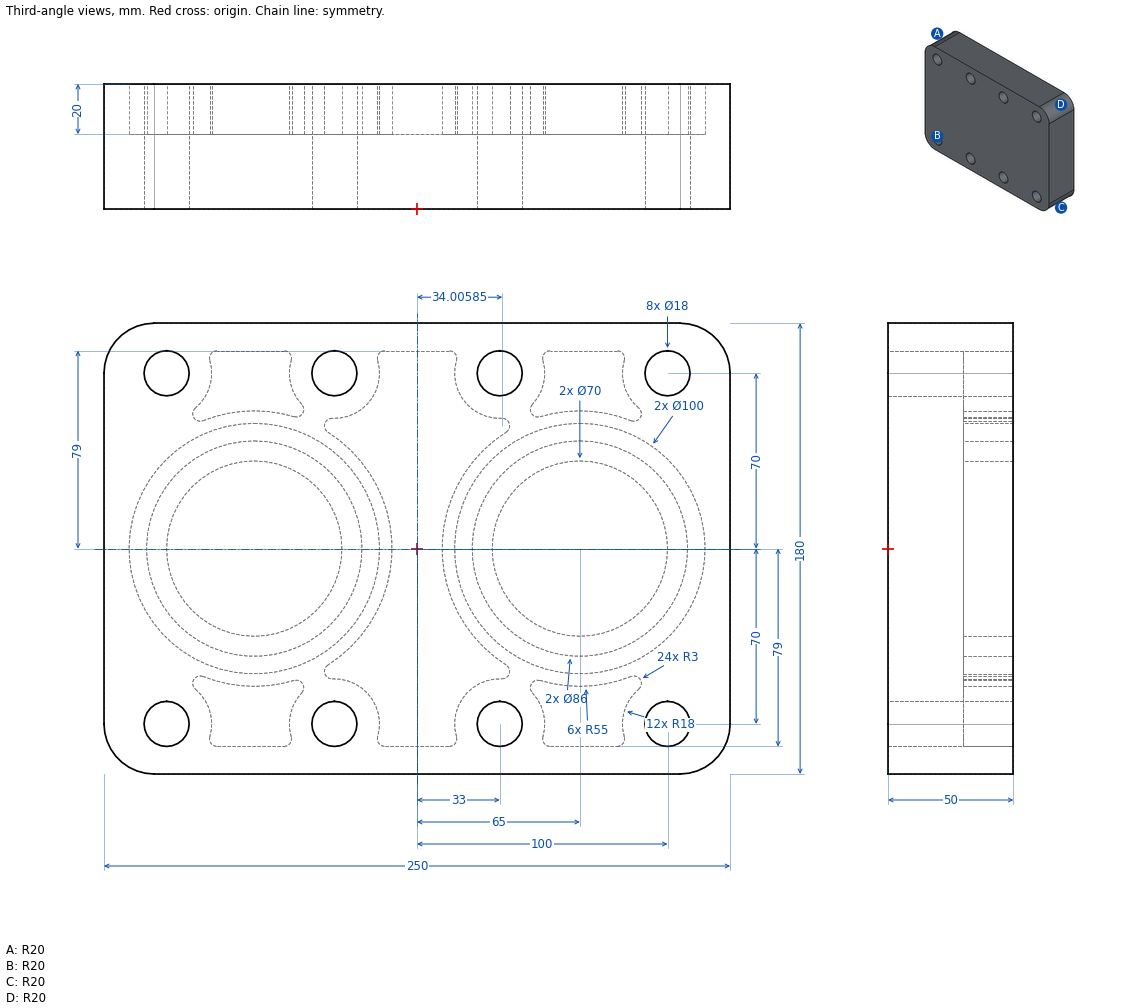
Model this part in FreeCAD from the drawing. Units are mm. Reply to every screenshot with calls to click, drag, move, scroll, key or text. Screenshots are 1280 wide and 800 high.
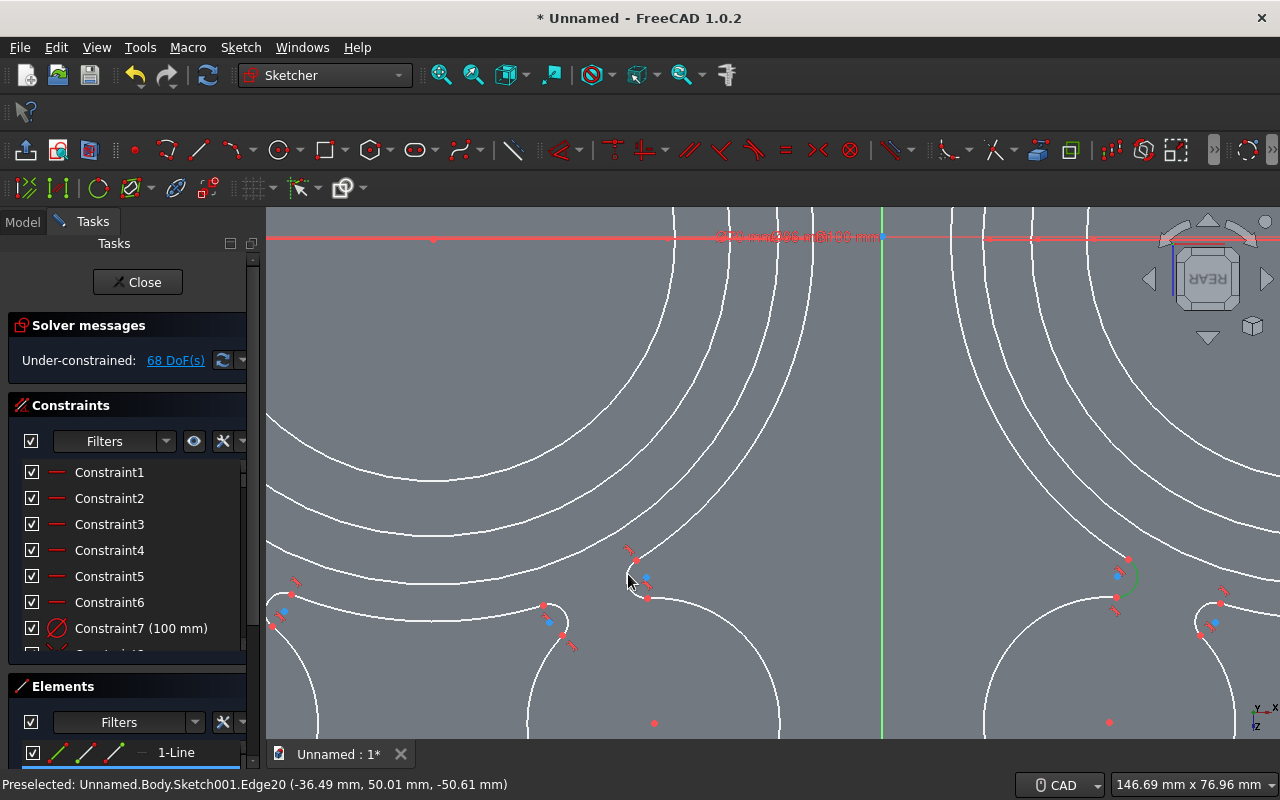
click(627, 574)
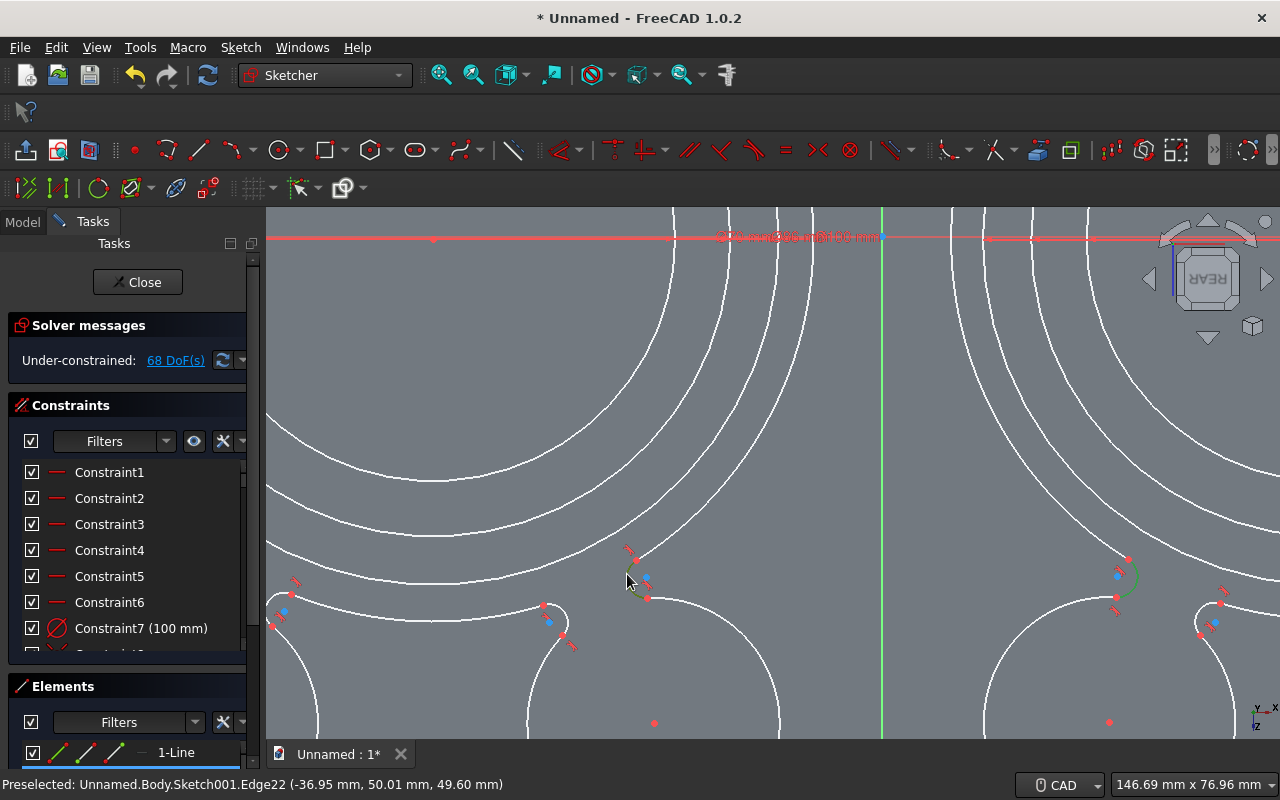
scroll(628, 575, down, 6)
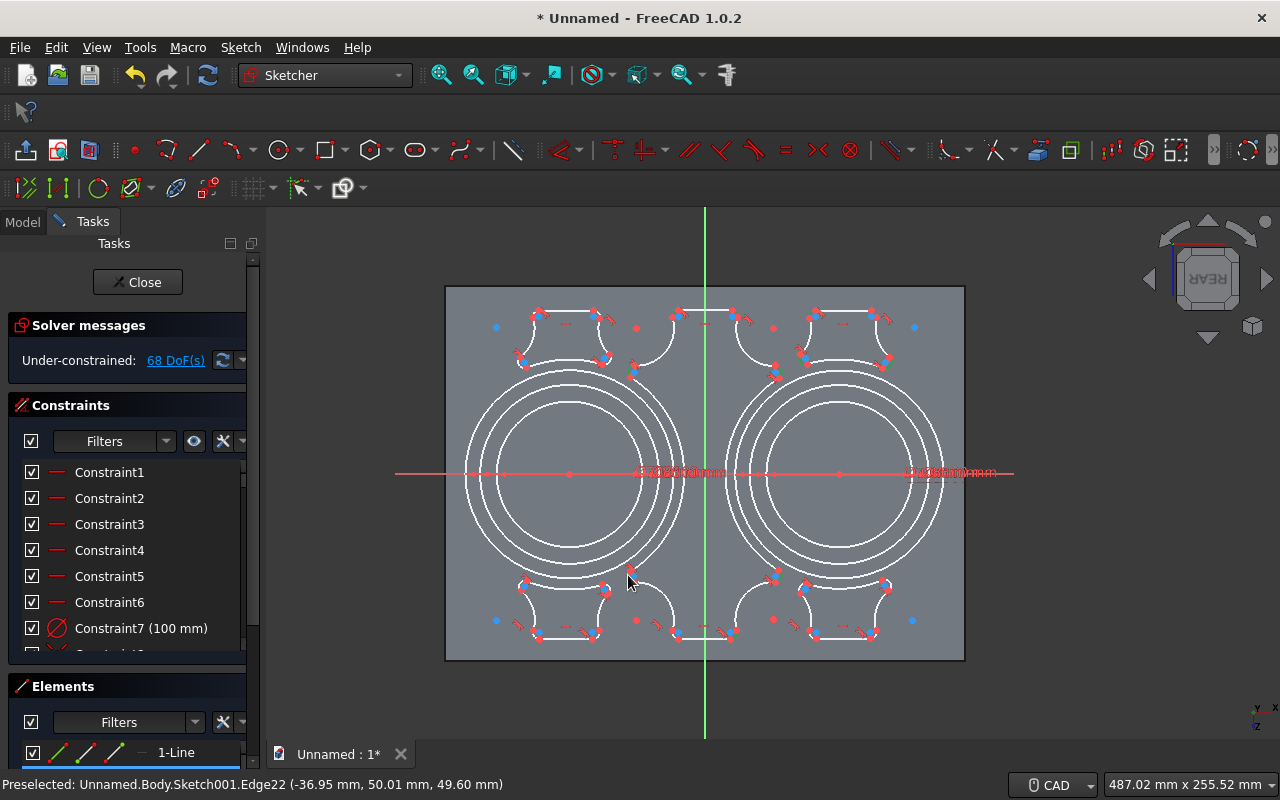
scroll(672, 634, up, 7)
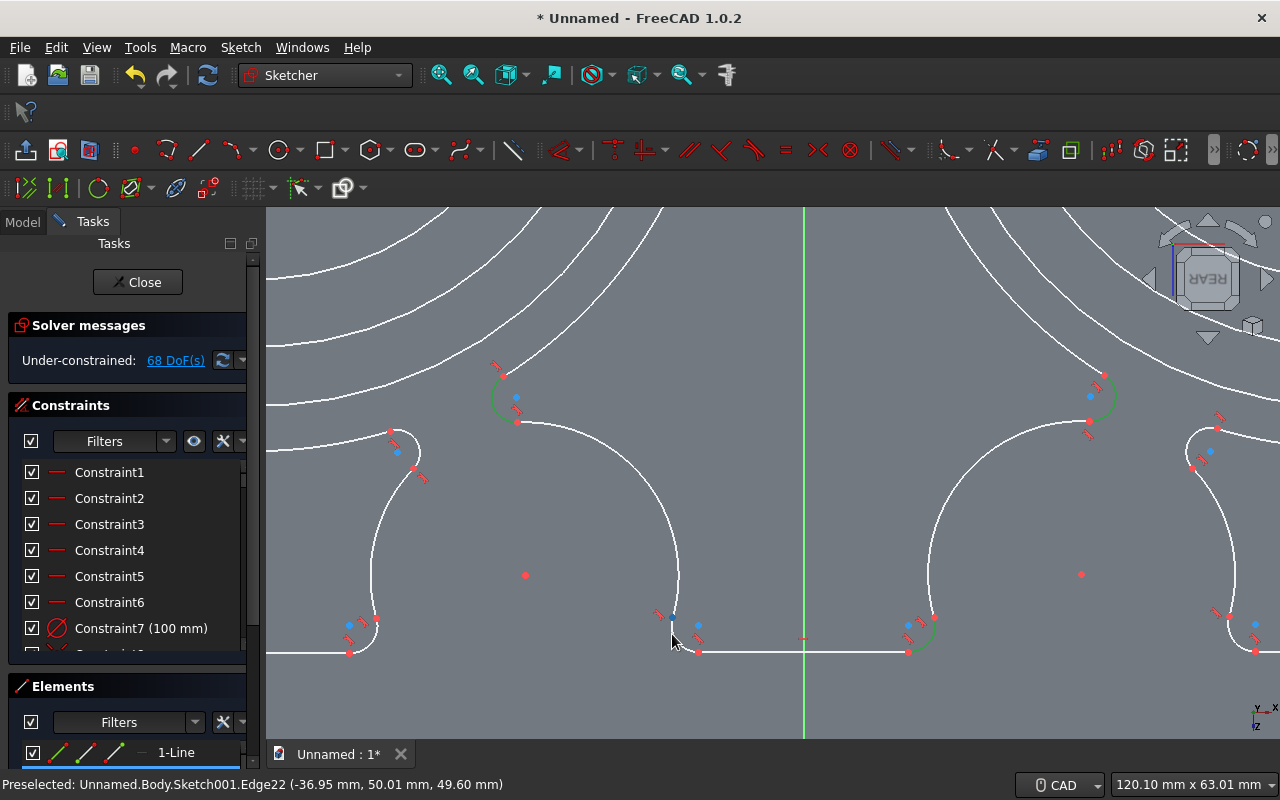
click(673, 633)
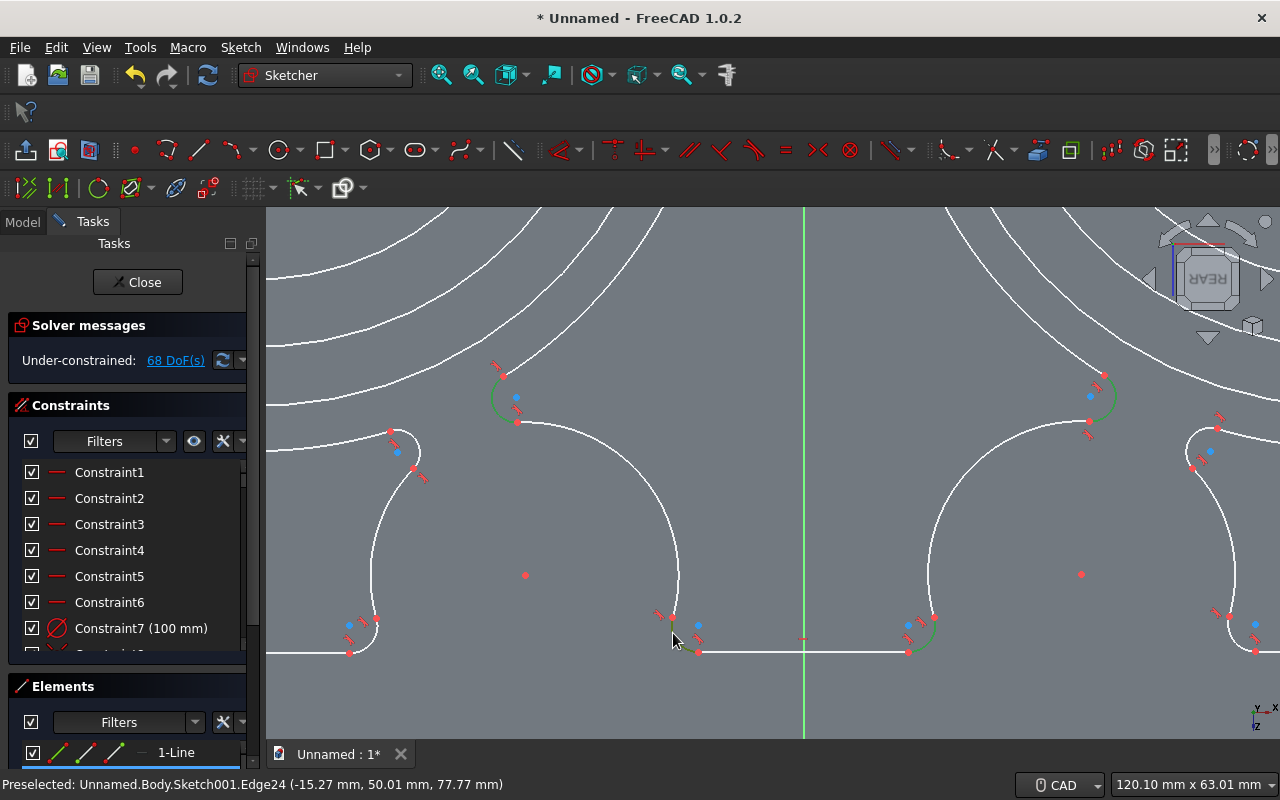
scroll(672, 634, down, 7)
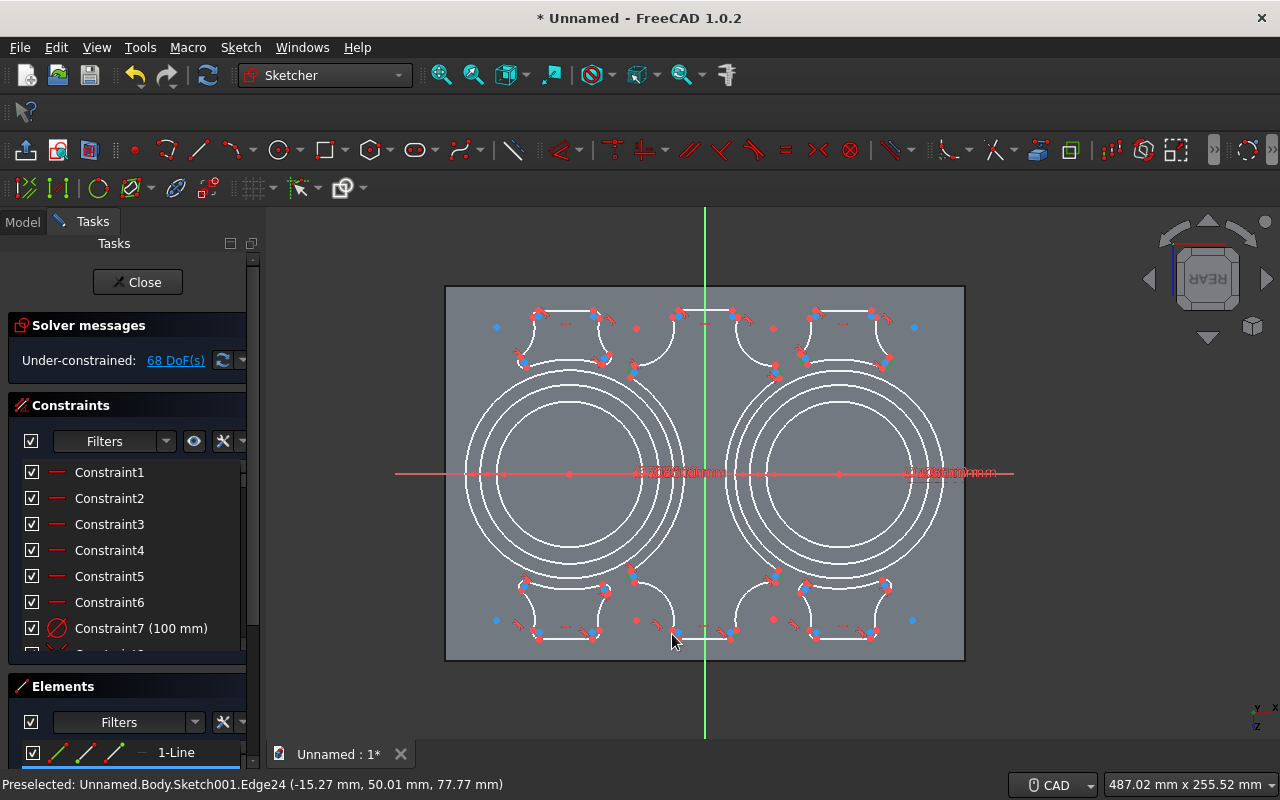
scroll(536, 311, up, 8)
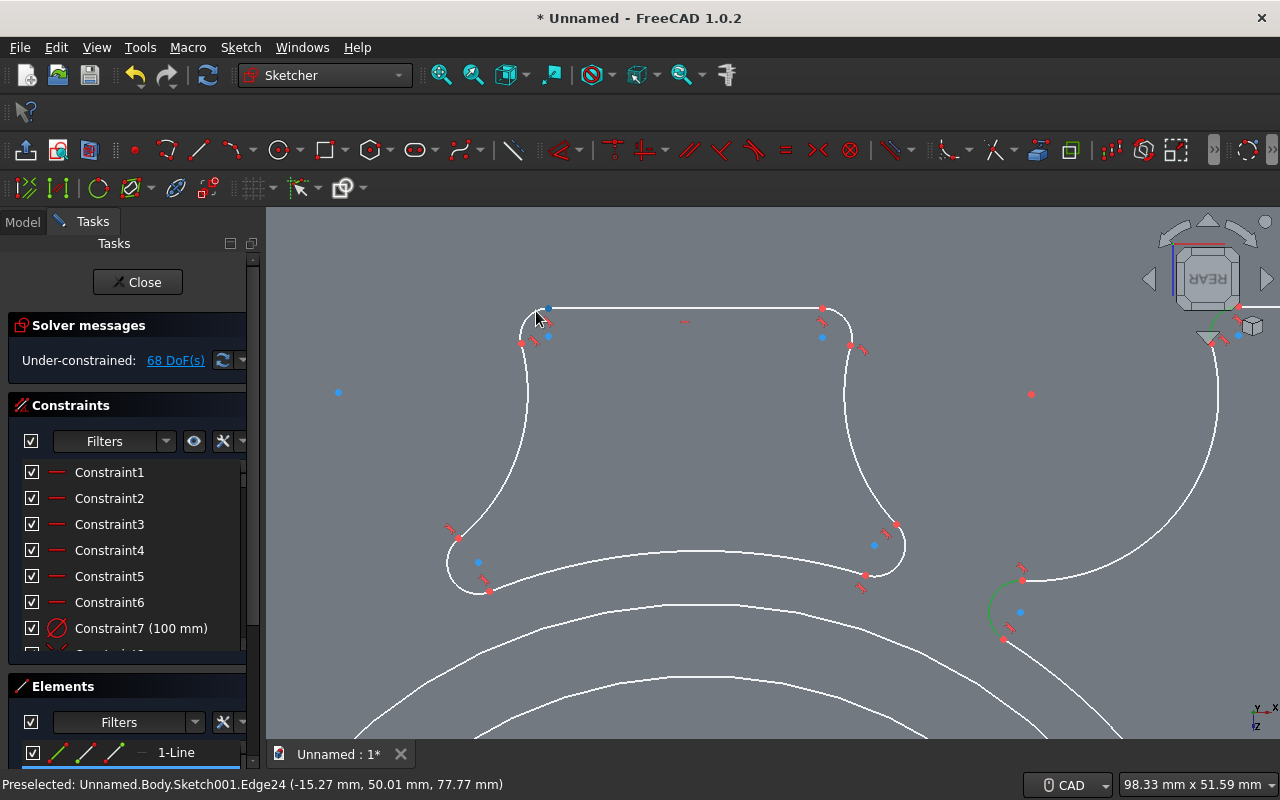
click(534, 312)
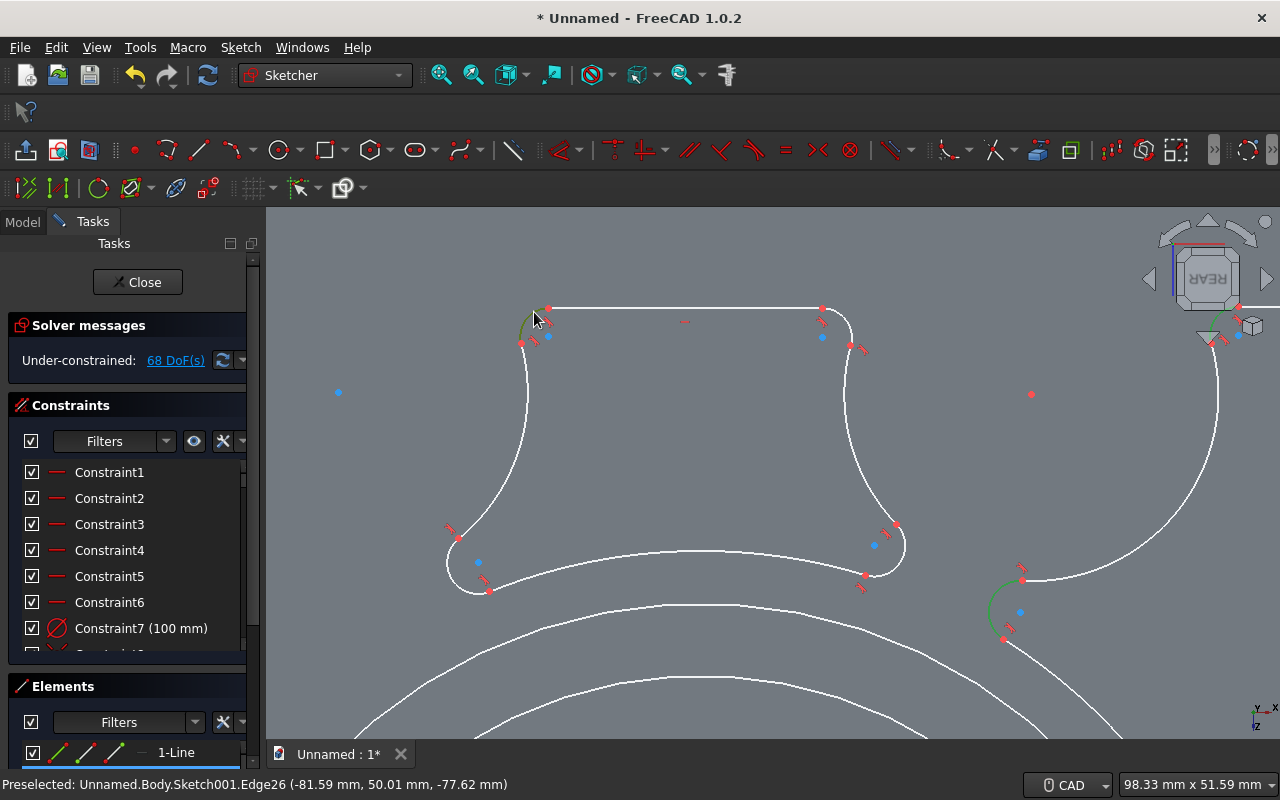
click(447, 562)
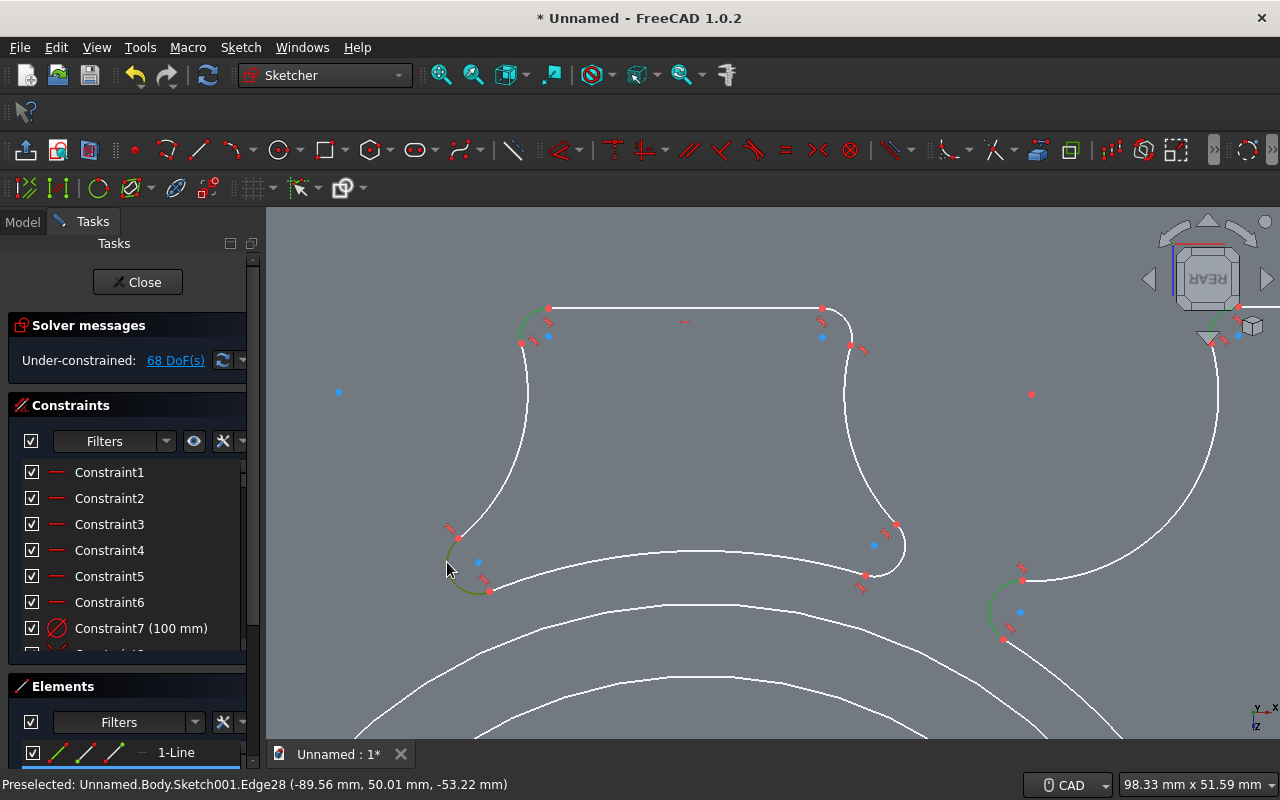
click(889, 573)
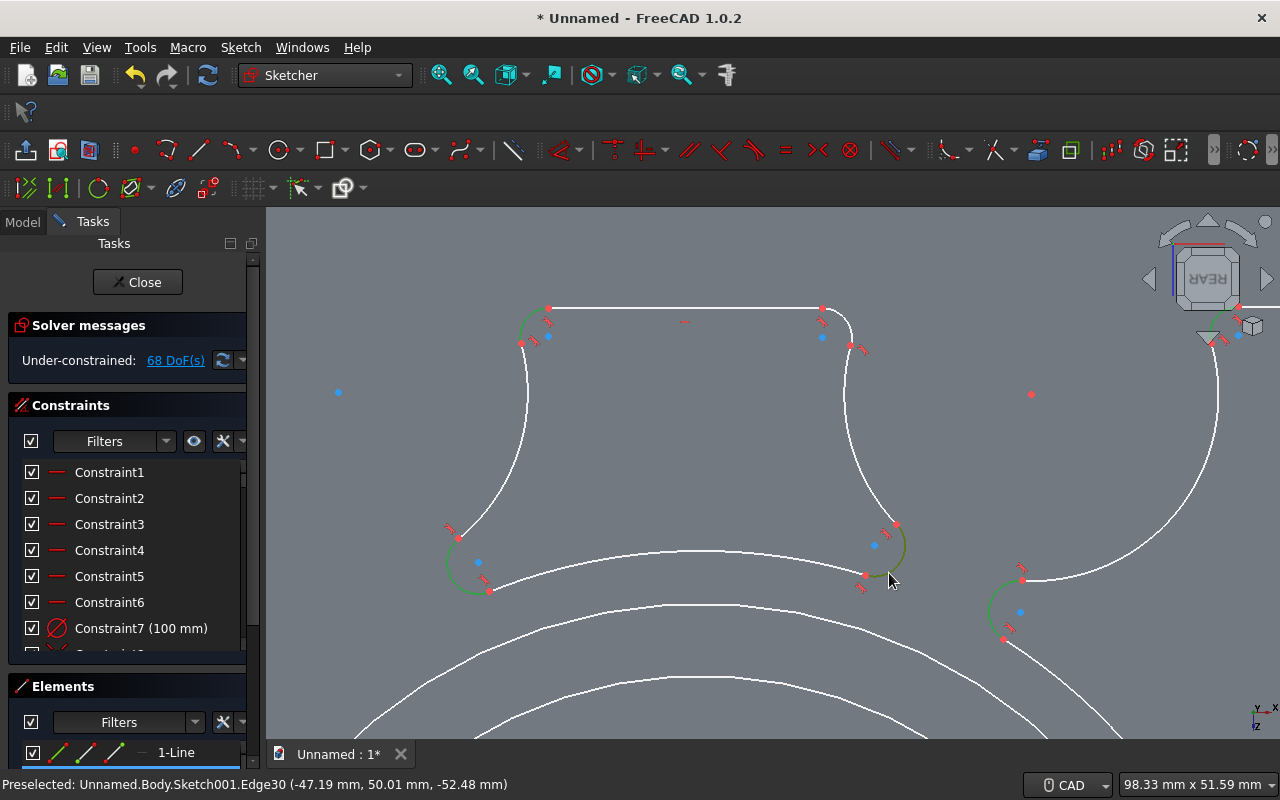
click(851, 330)